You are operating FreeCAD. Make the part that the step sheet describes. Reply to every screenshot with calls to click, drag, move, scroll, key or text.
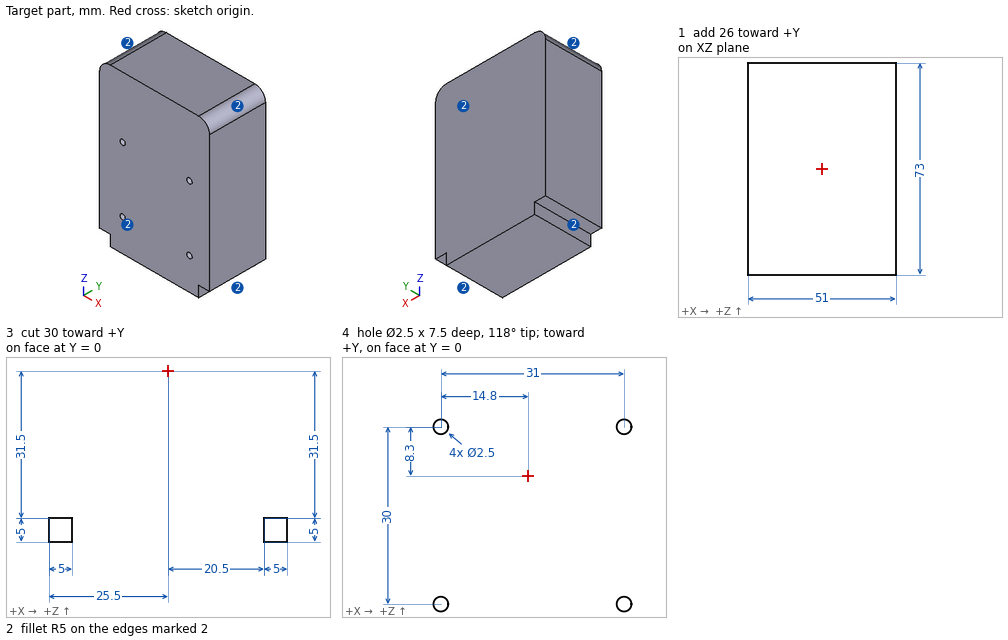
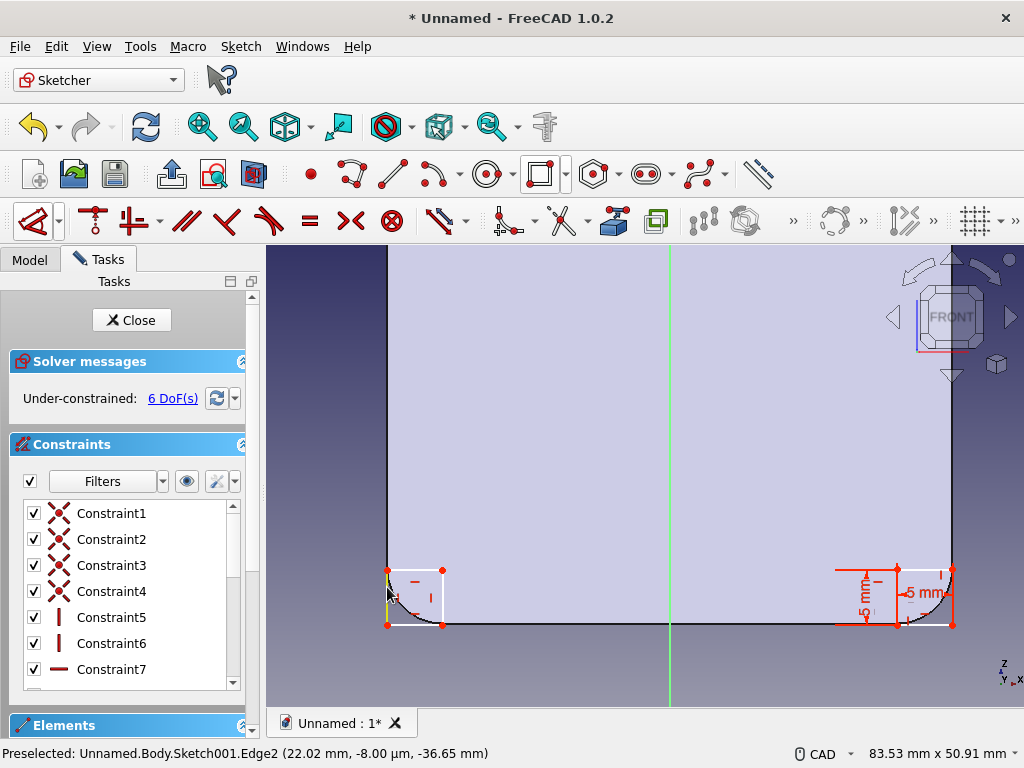
click(387, 587)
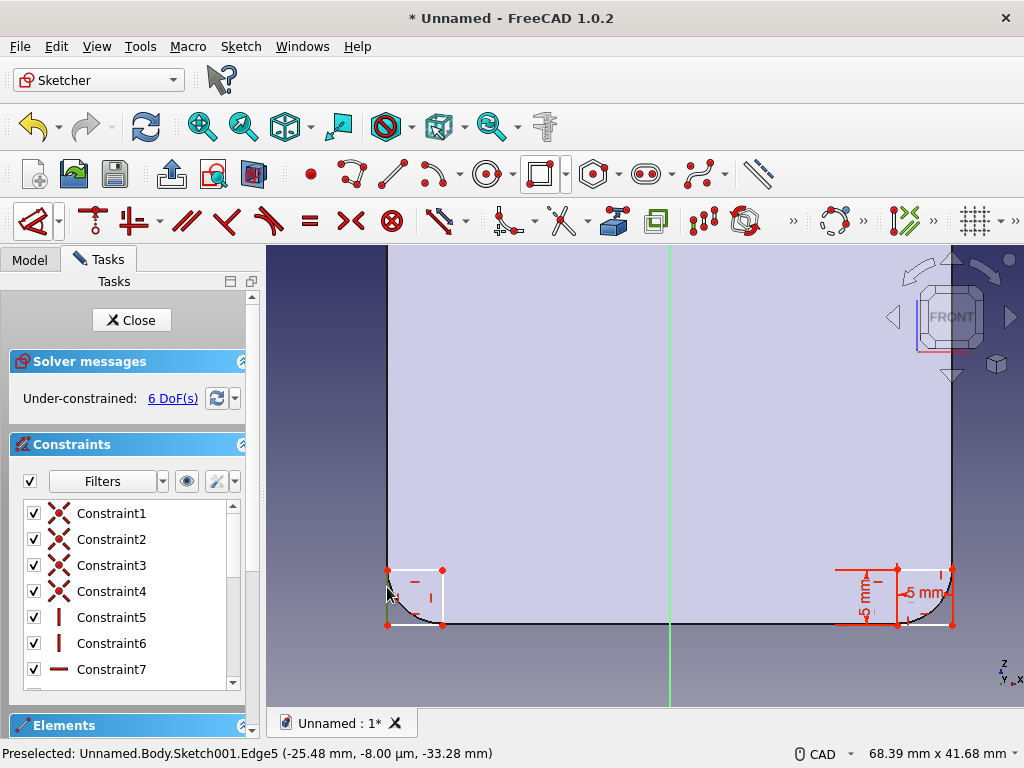
key(i)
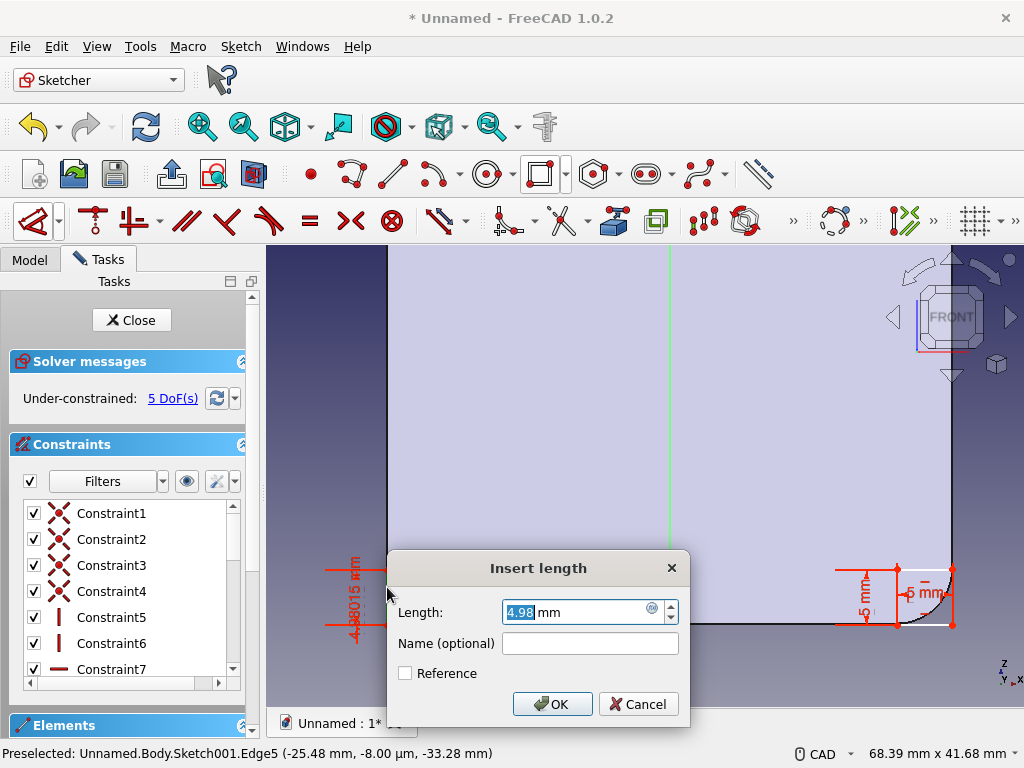
text(5)
key(Return)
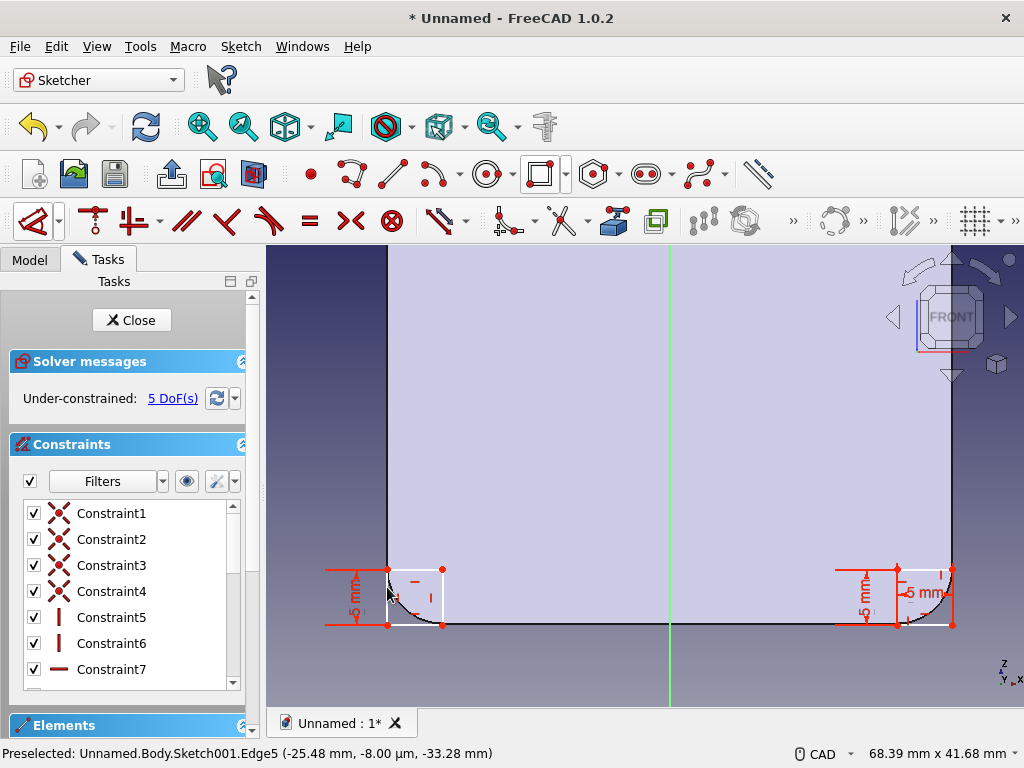
click(404, 625)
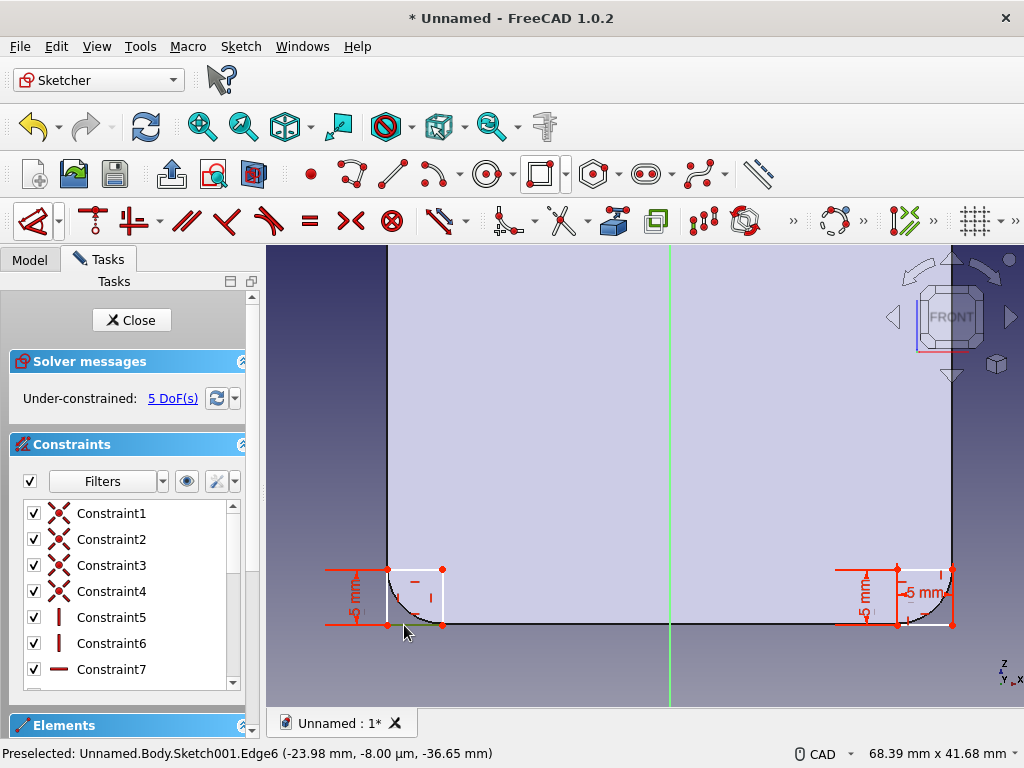
key(l)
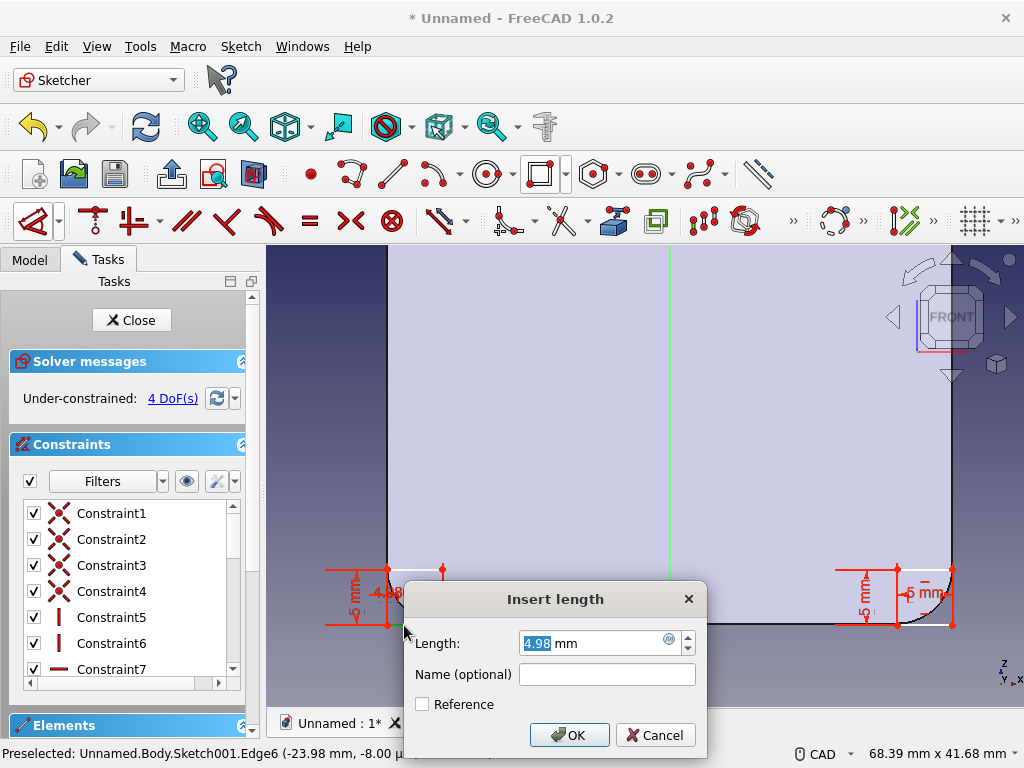
text(5)
key(Return)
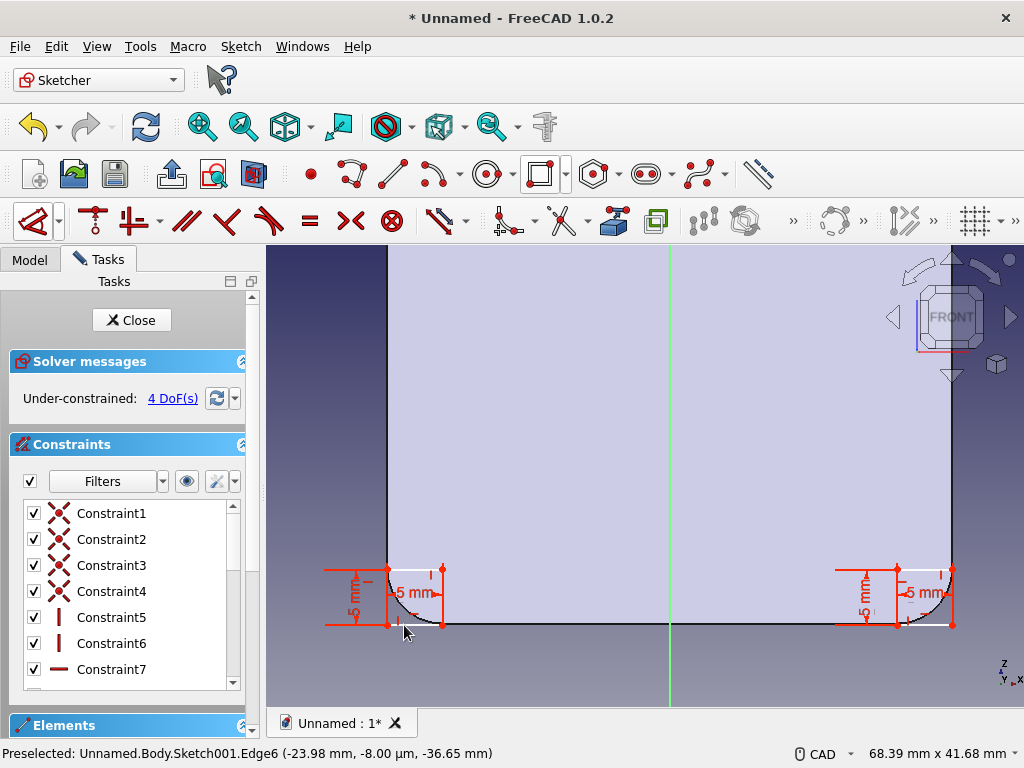
scroll(387, 587, down, 2)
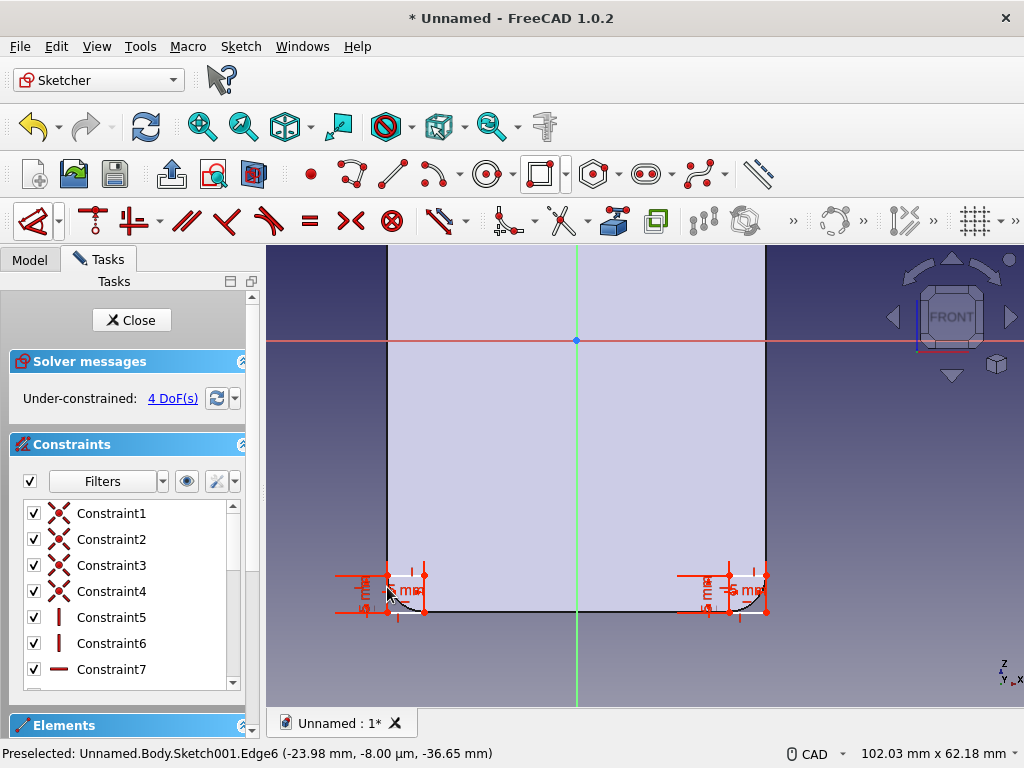
click(729, 576)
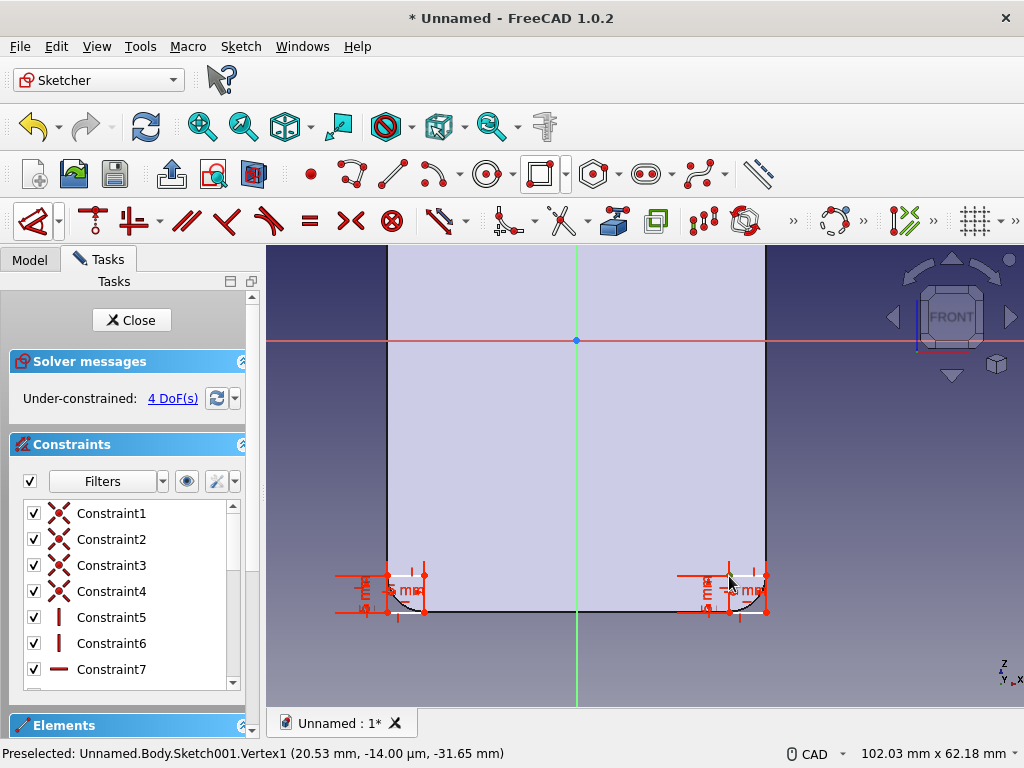
key(l)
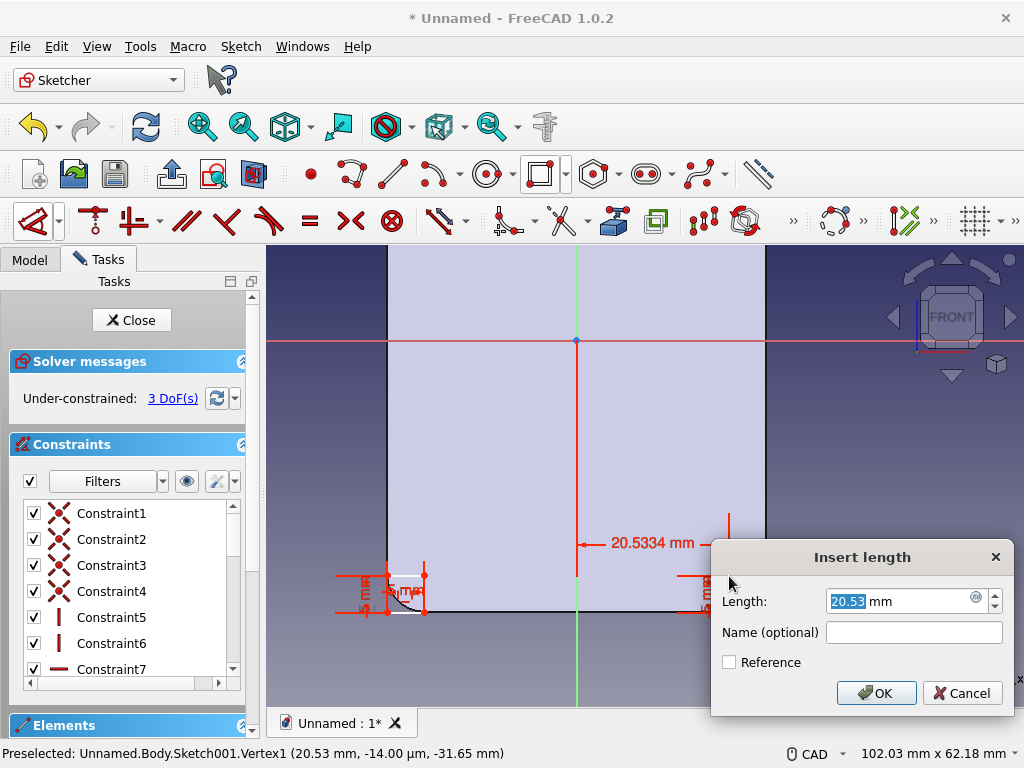
text(20.5)
key(Return)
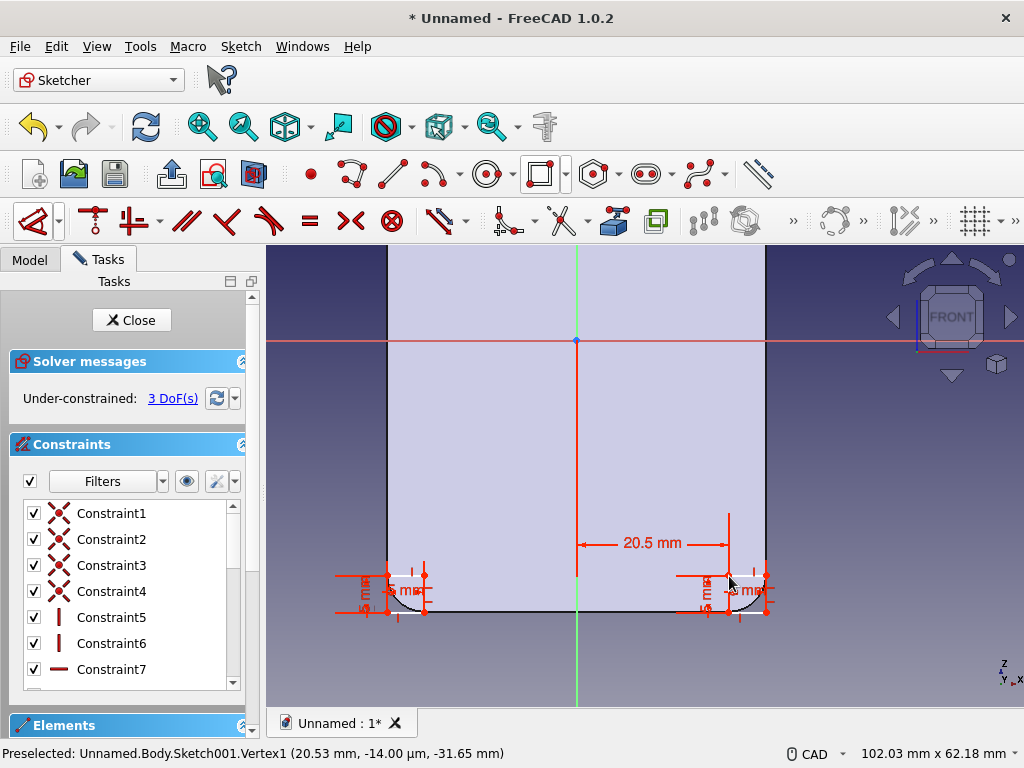
click(729, 576)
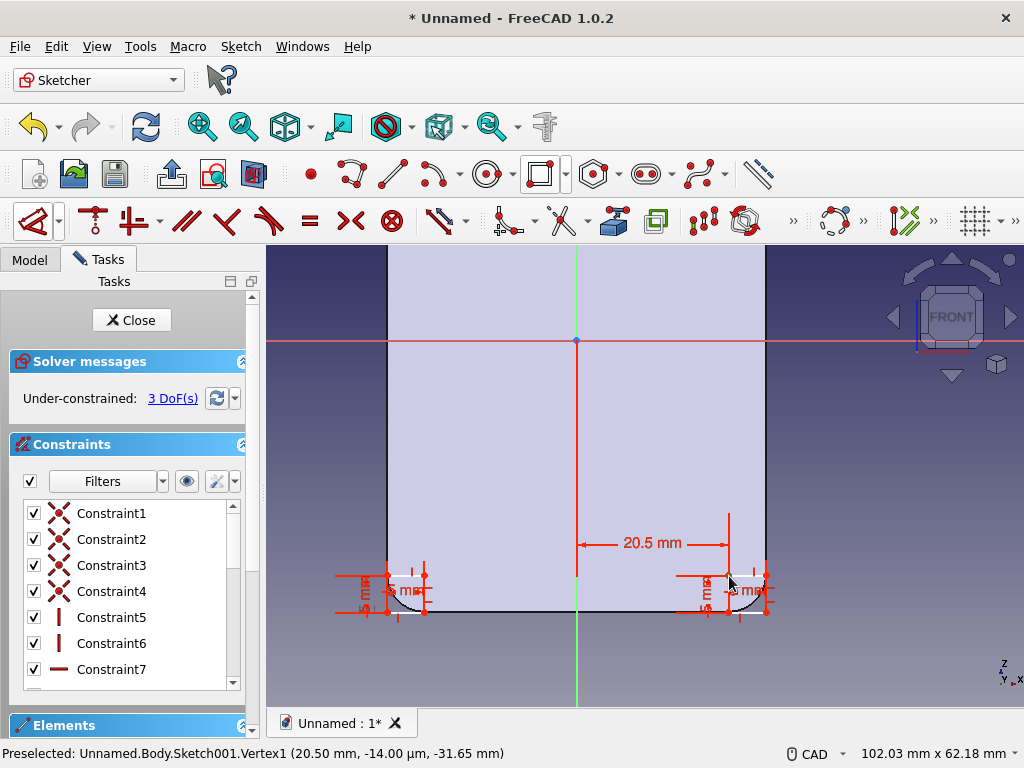
click(58, 222)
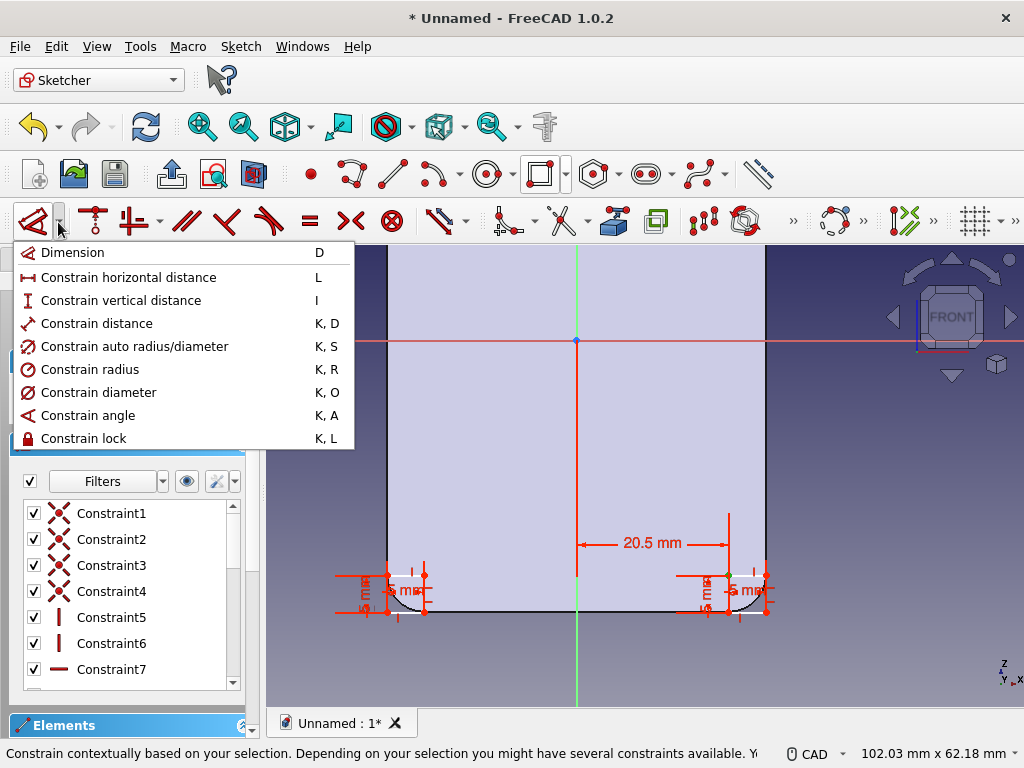
click(184, 300)